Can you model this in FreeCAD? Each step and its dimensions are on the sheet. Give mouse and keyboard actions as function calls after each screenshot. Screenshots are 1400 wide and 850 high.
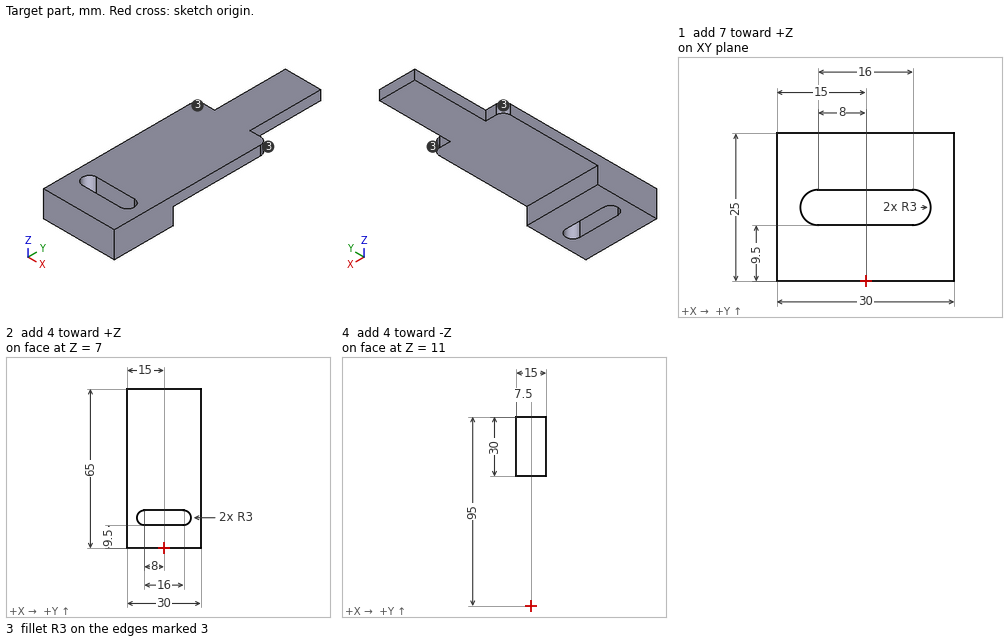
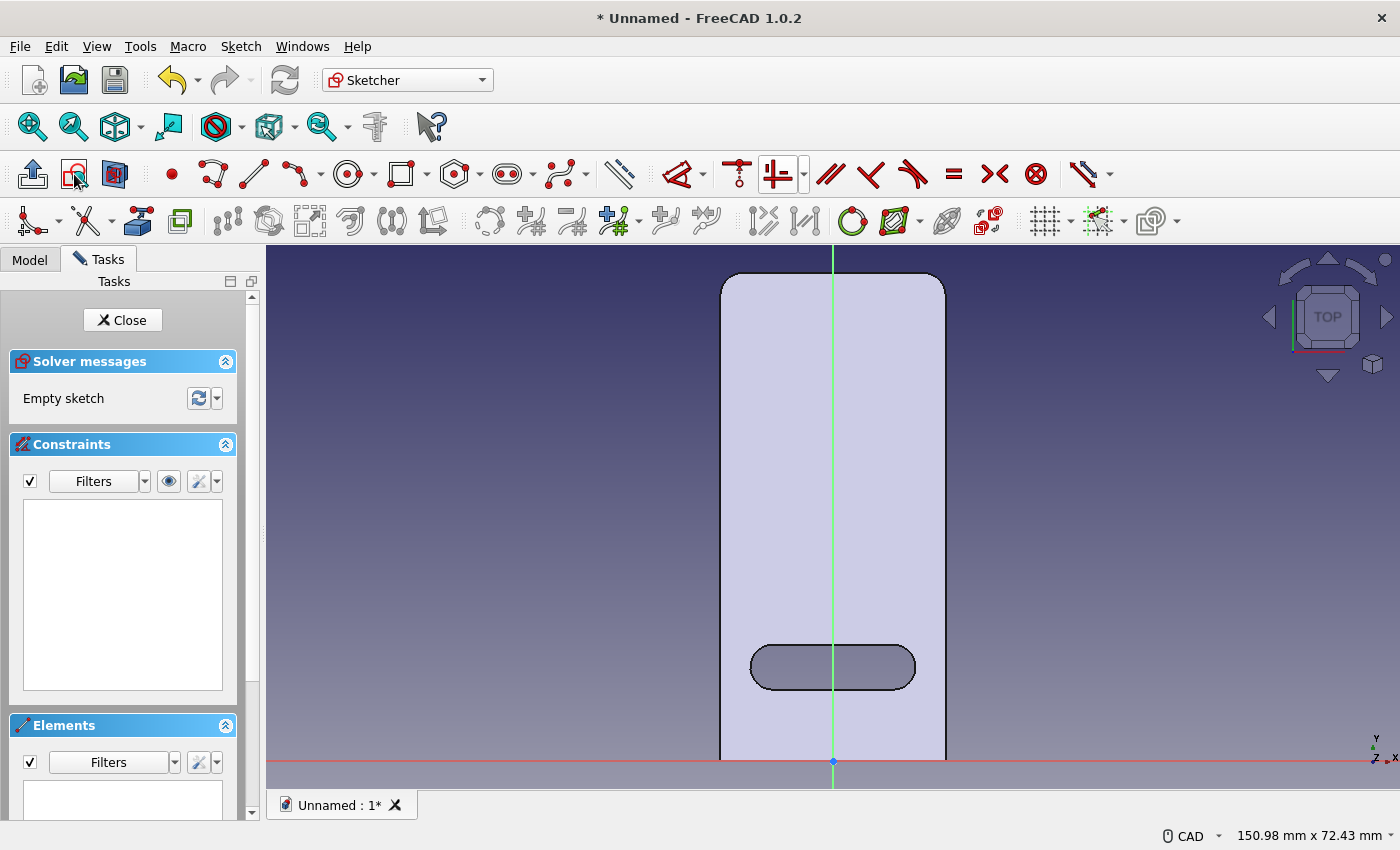
scroll(764, 517, down, 5)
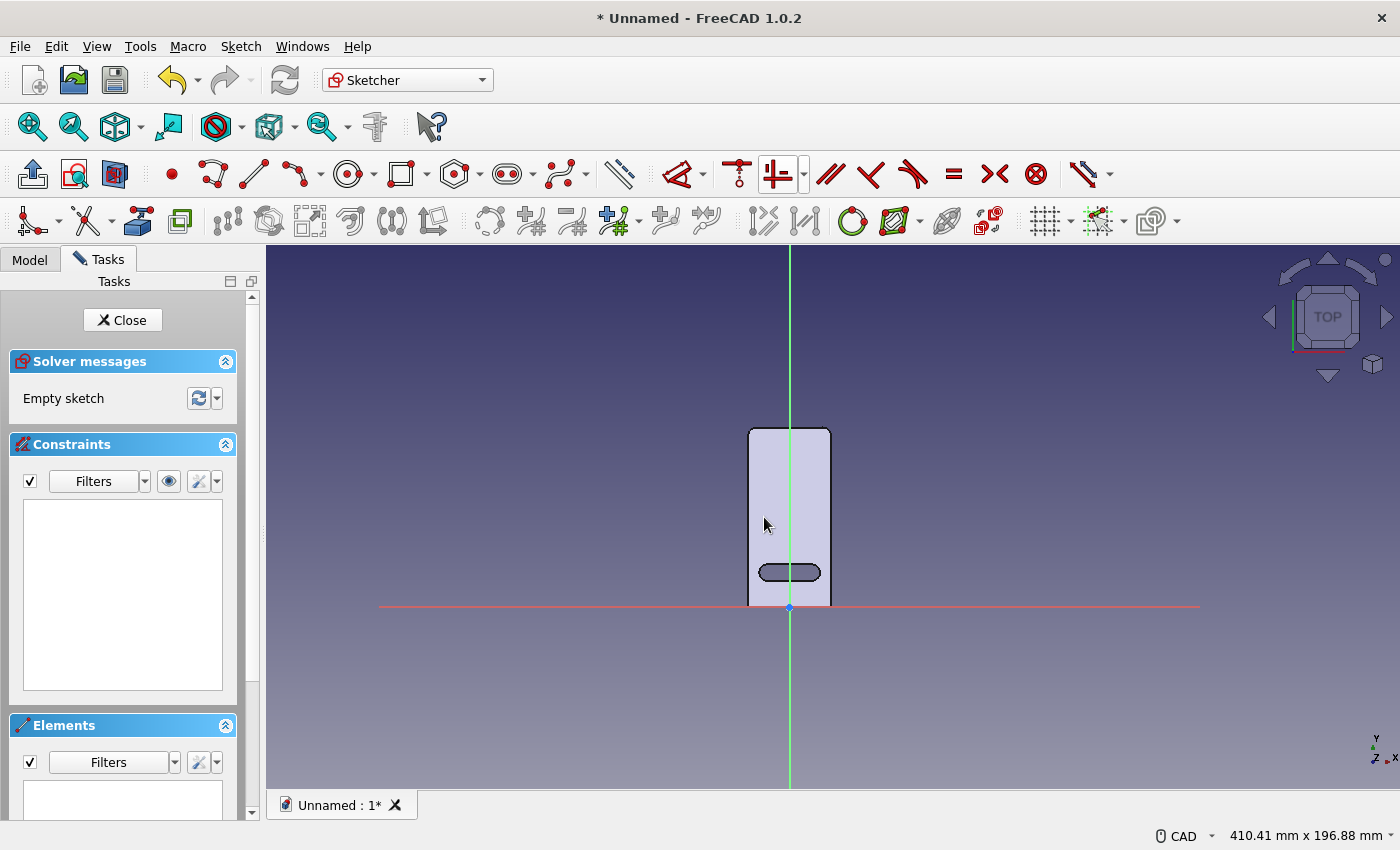
scroll(798, 343, up, 7)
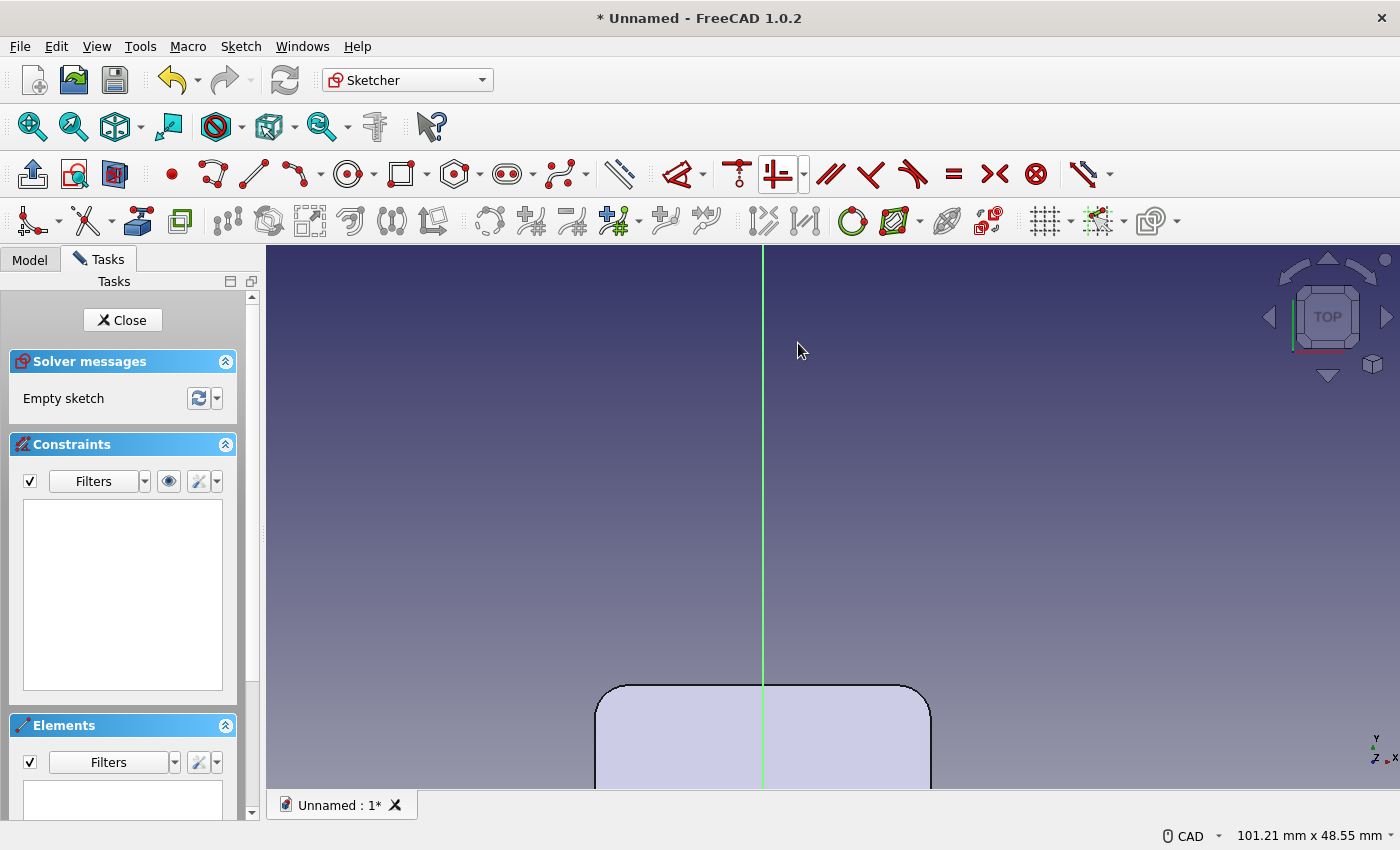
click(400, 174)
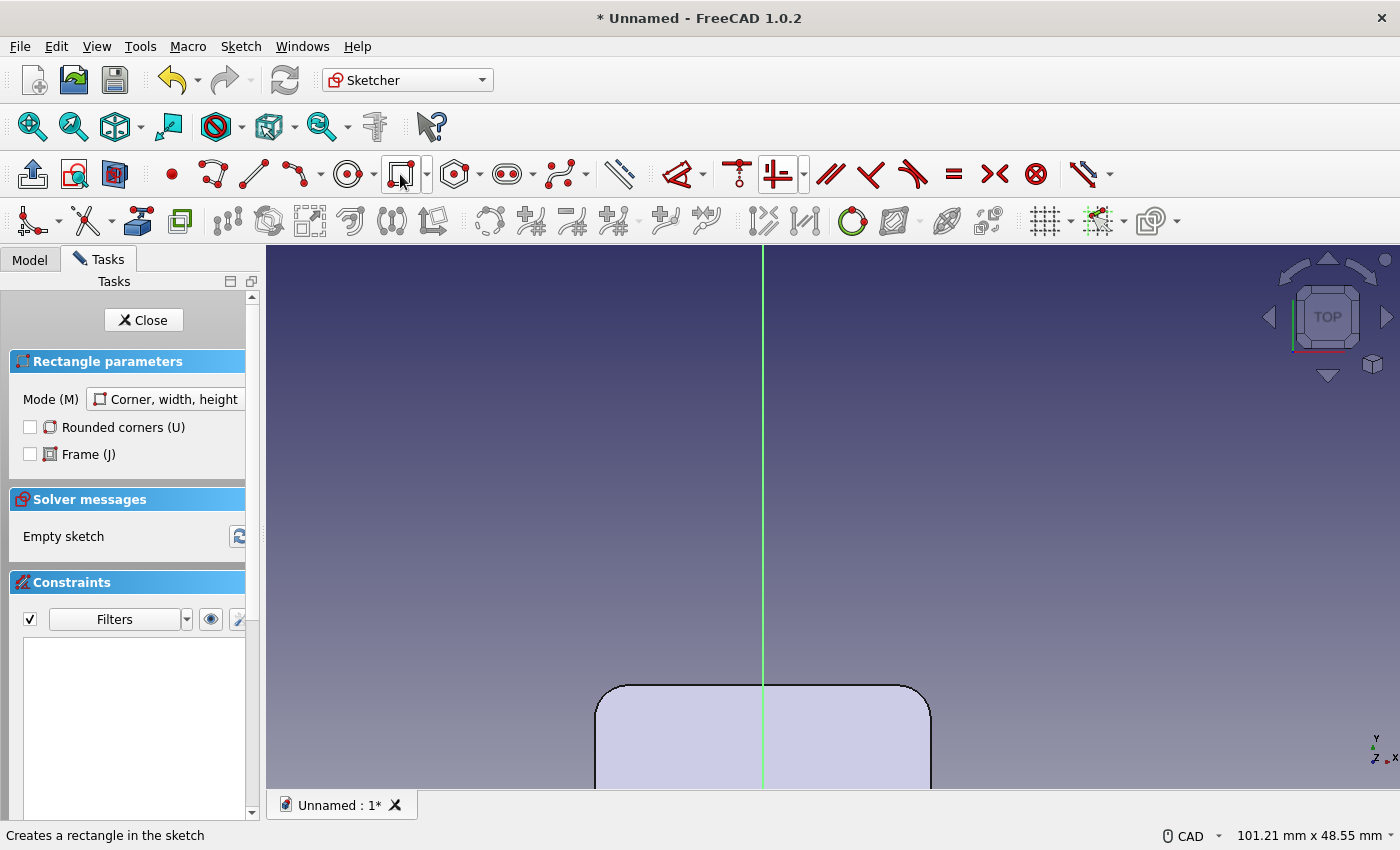
click(679, 349)
click(847, 685)
key(Escape)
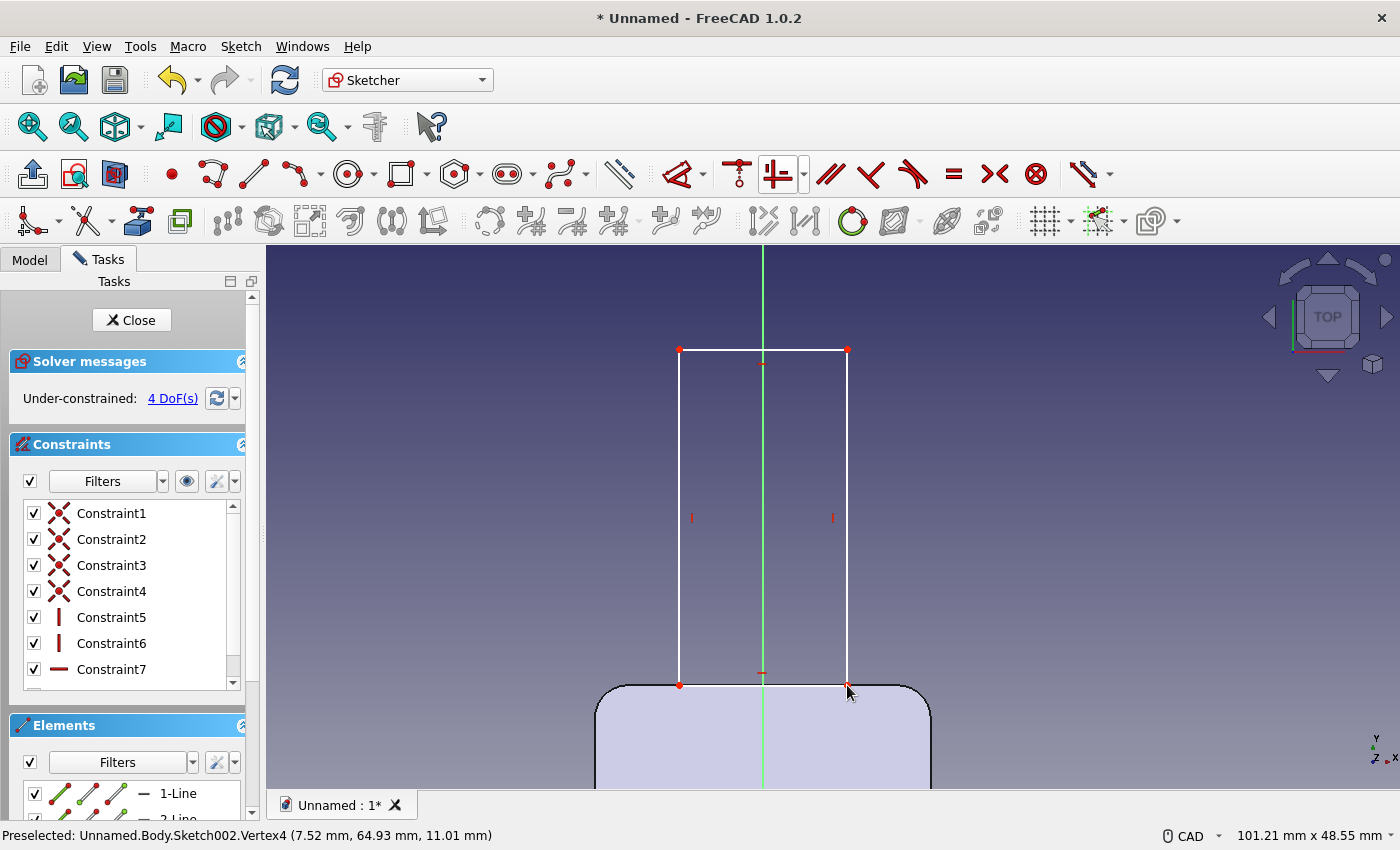
click(676, 174)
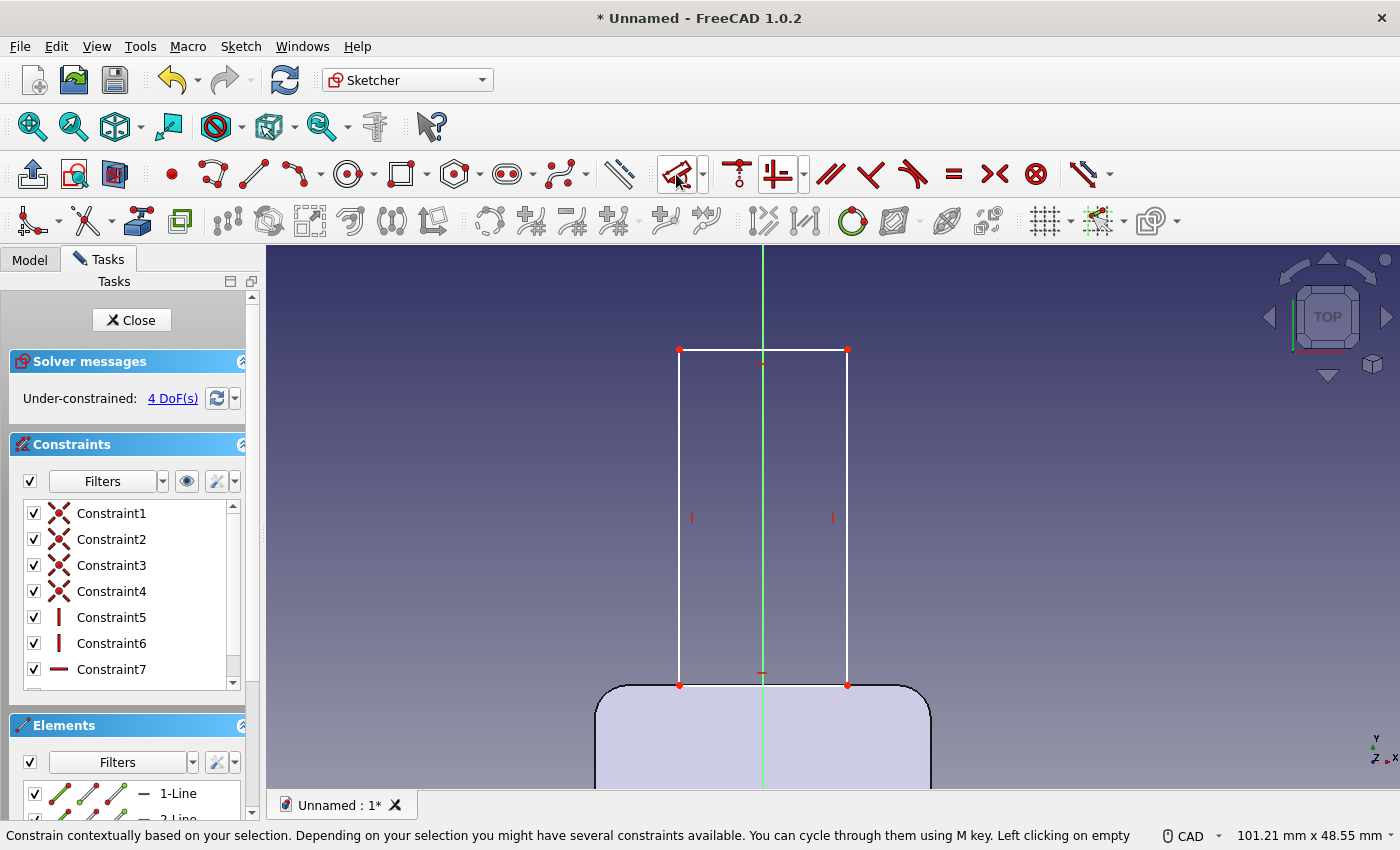
click(679, 451)
click(645, 518)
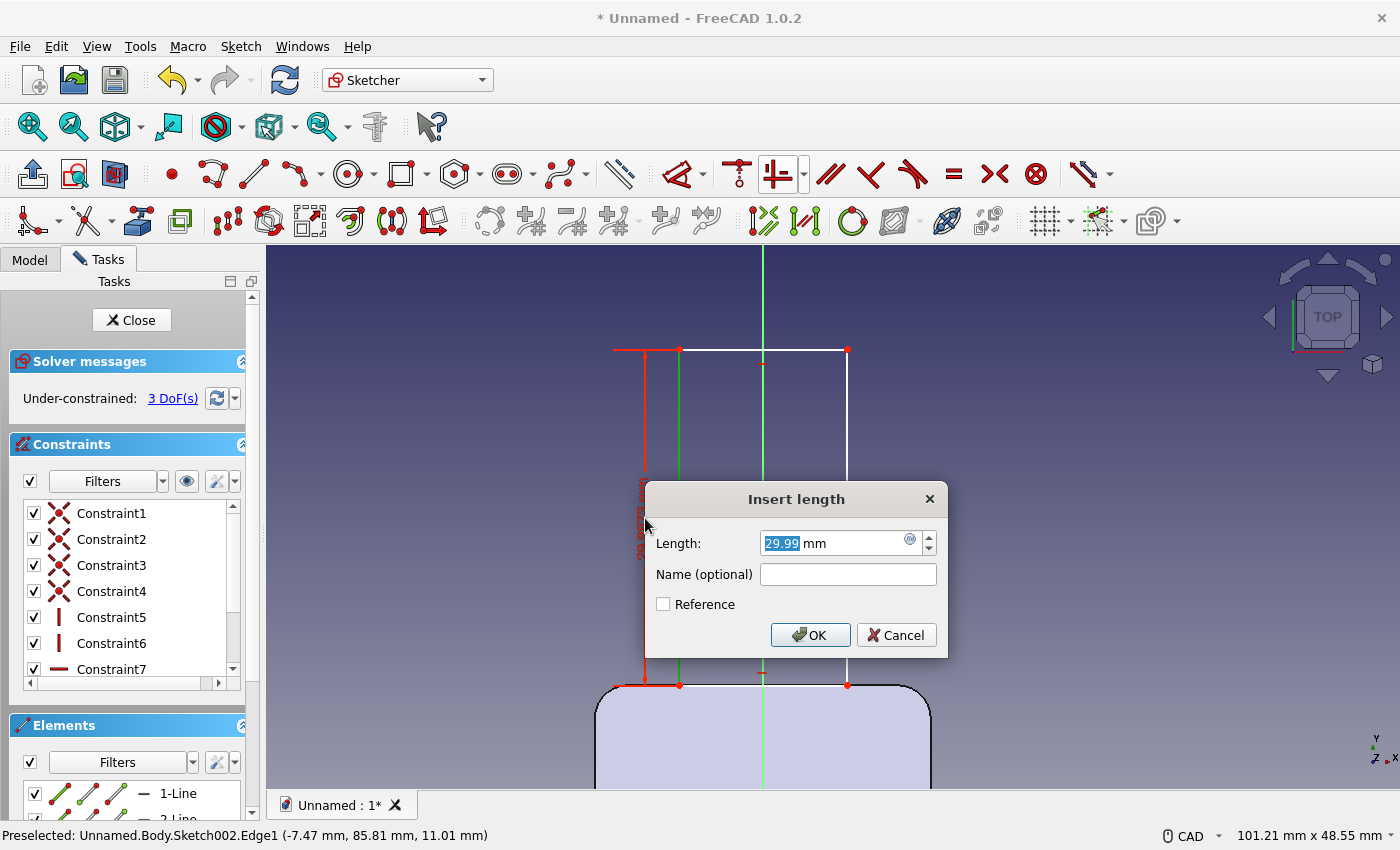
text(30)
key(Return)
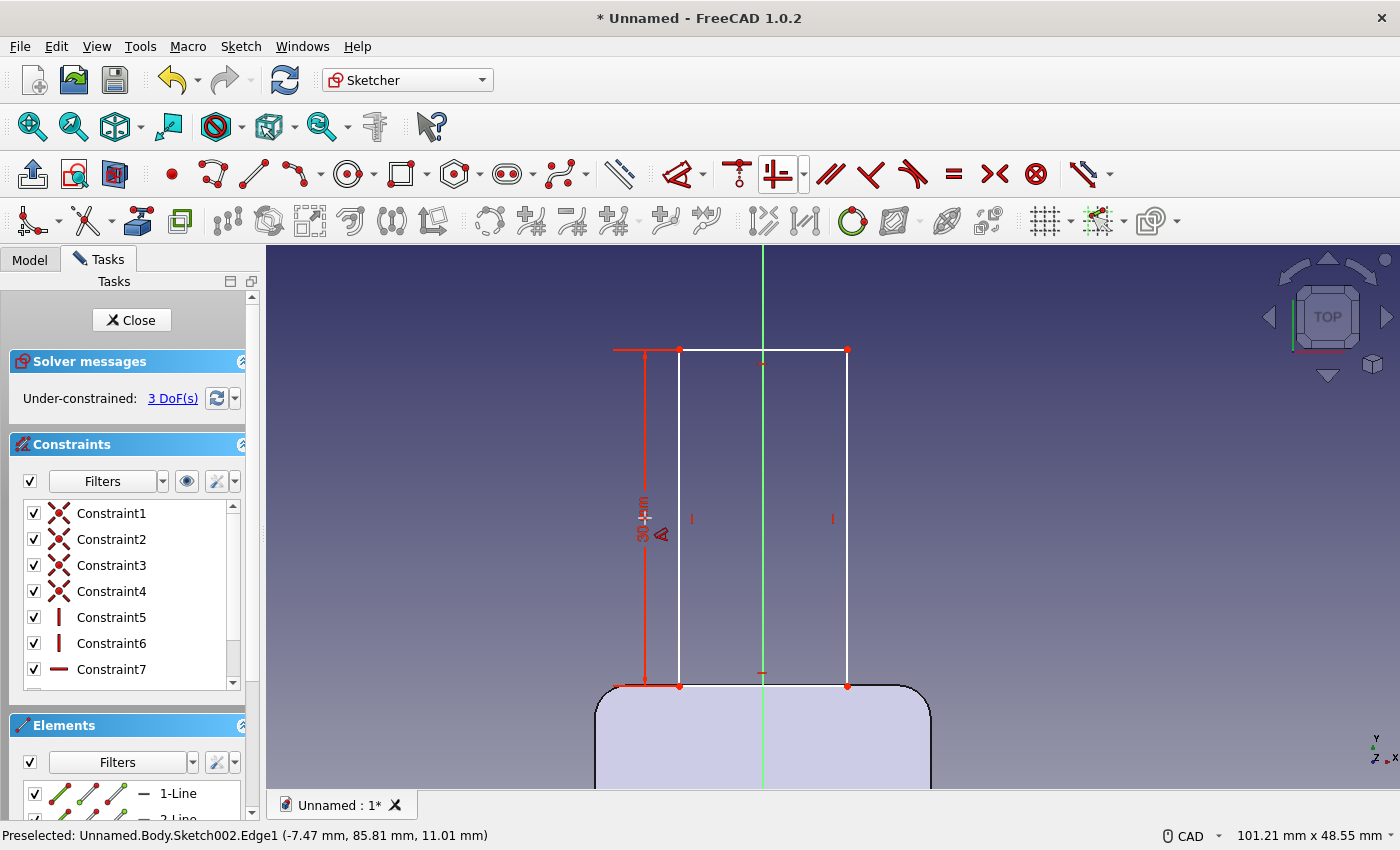
click(729, 686)
click(724, 720)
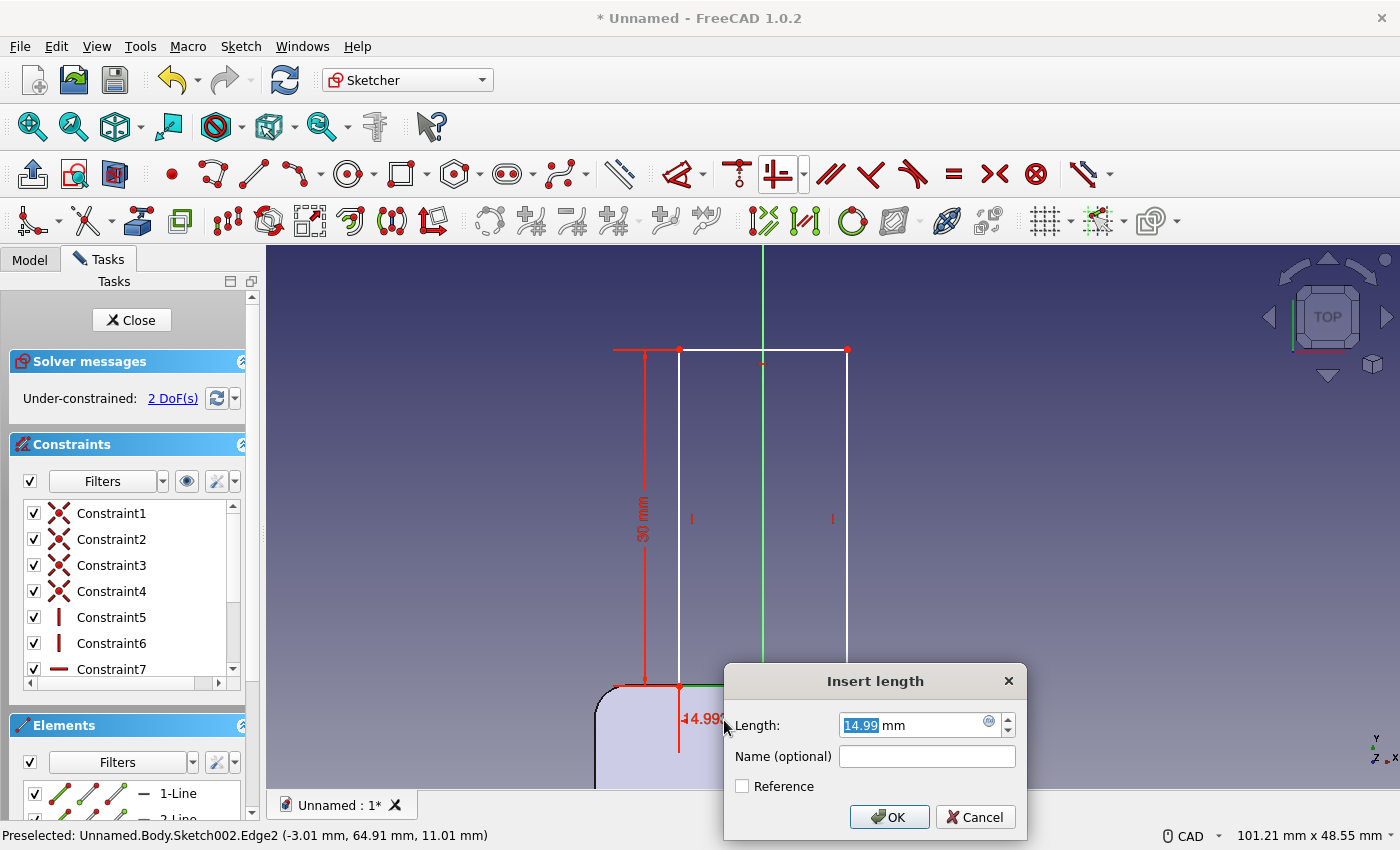
text(15)
key(Return)